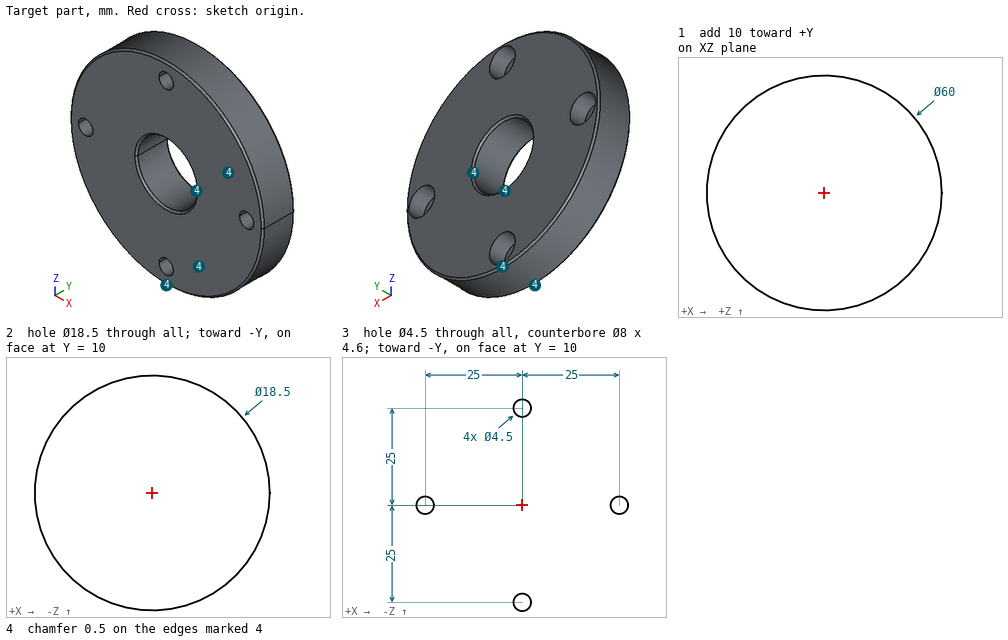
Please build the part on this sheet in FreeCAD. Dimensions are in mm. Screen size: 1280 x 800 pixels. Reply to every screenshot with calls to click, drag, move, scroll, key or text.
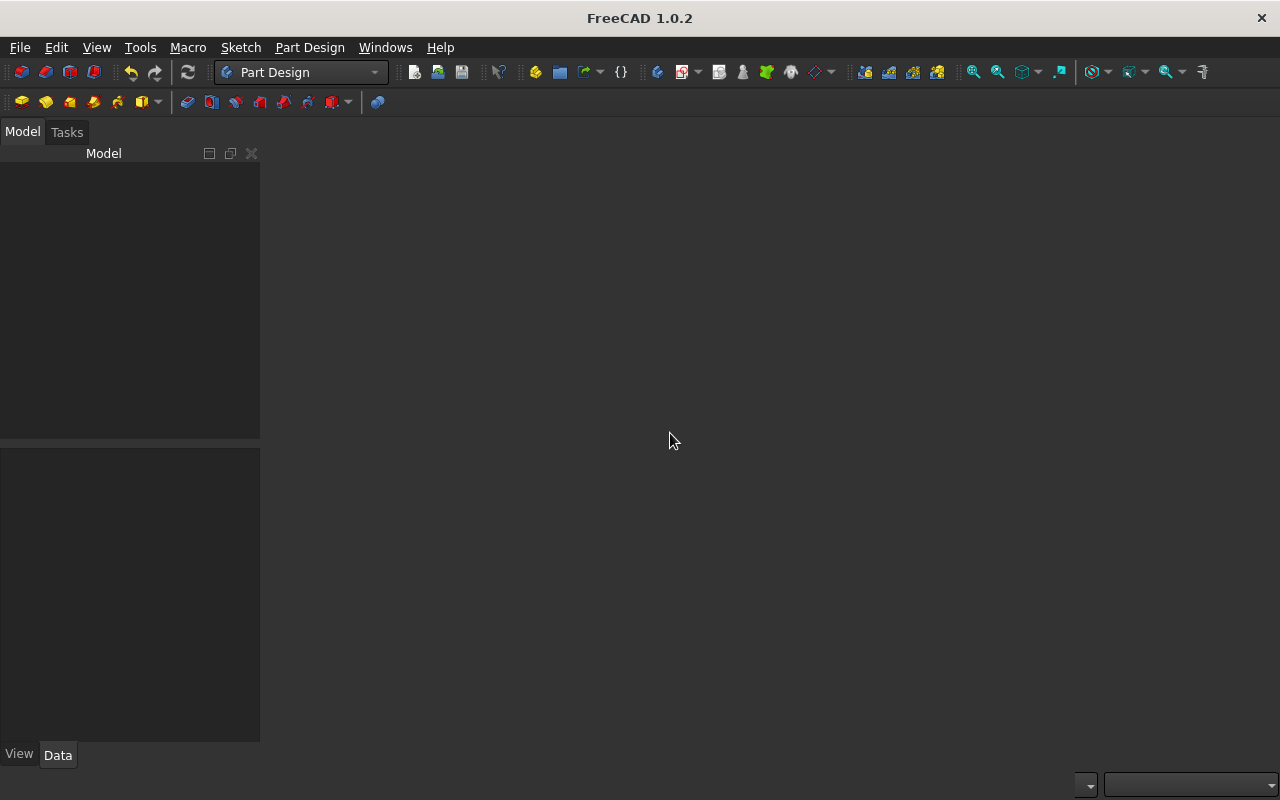
key(ctrl+n)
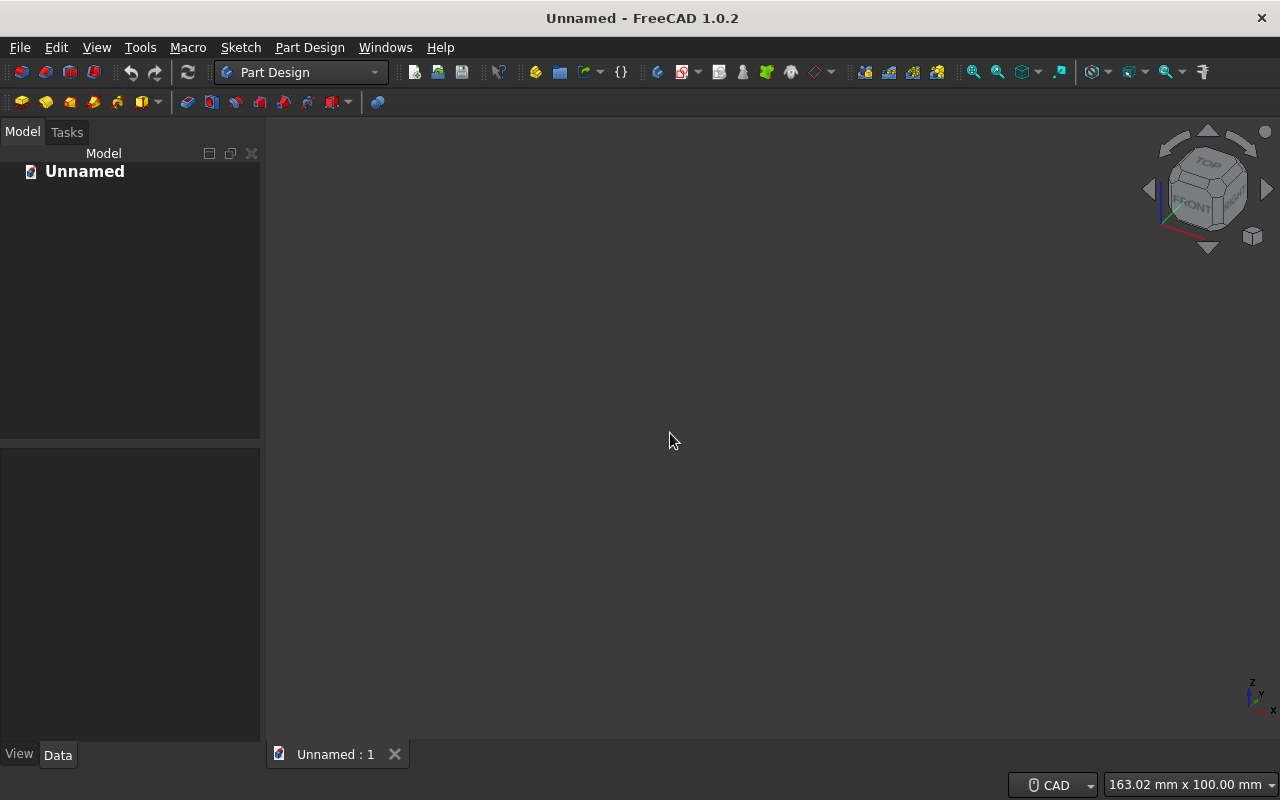
click(682, 72)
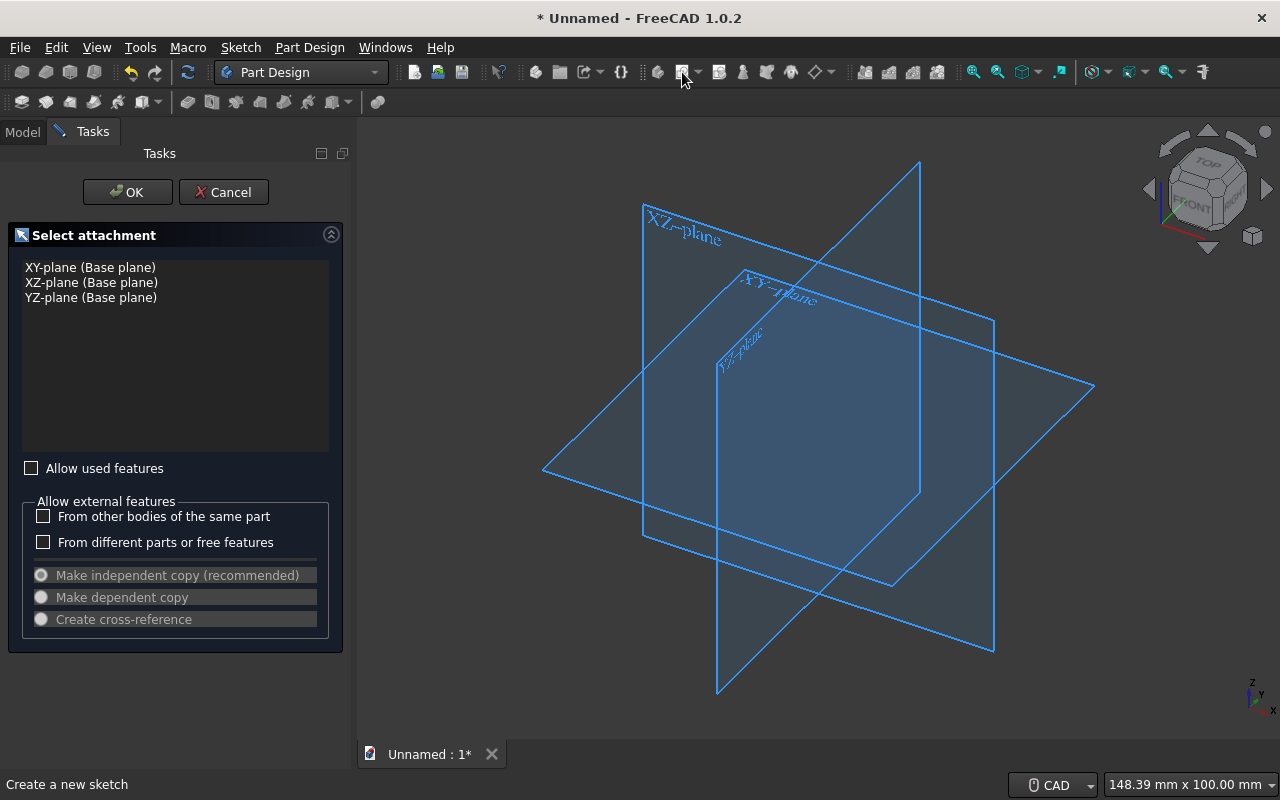
click(82, 282)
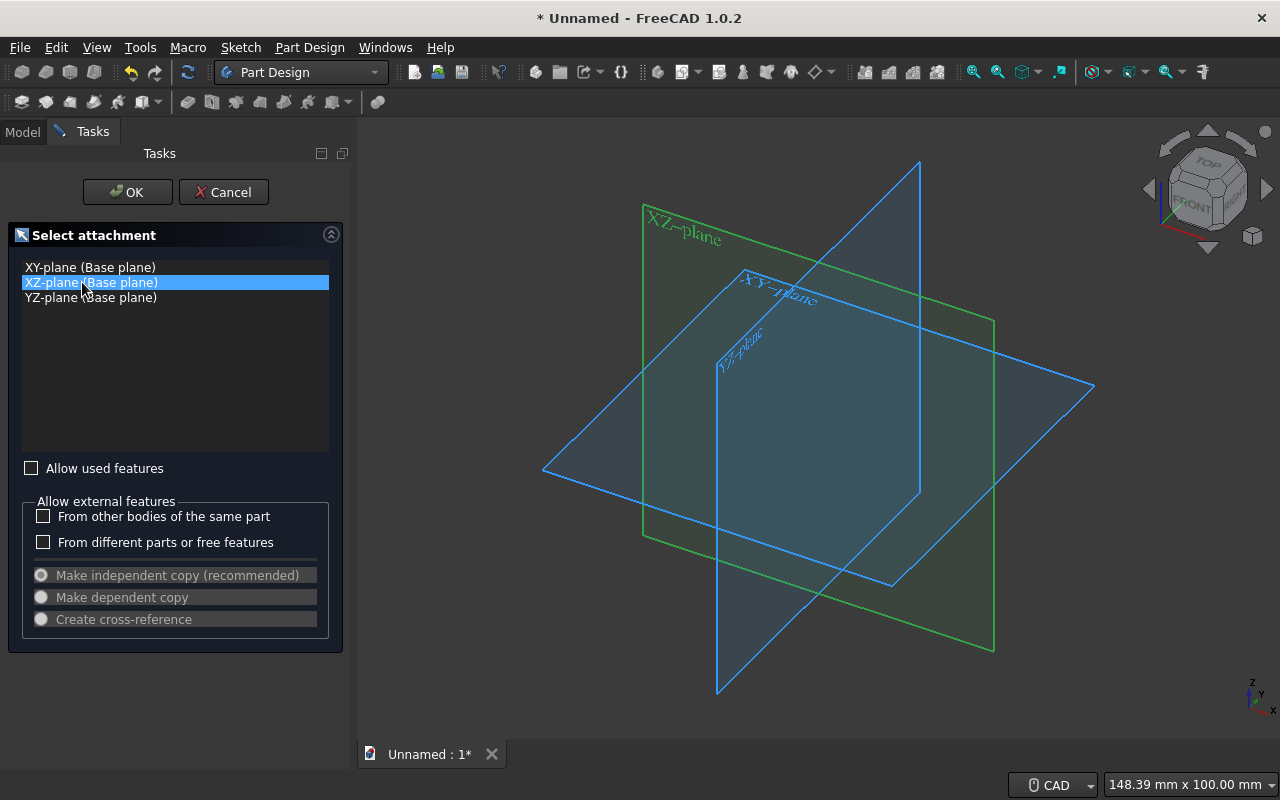
click(128, 192)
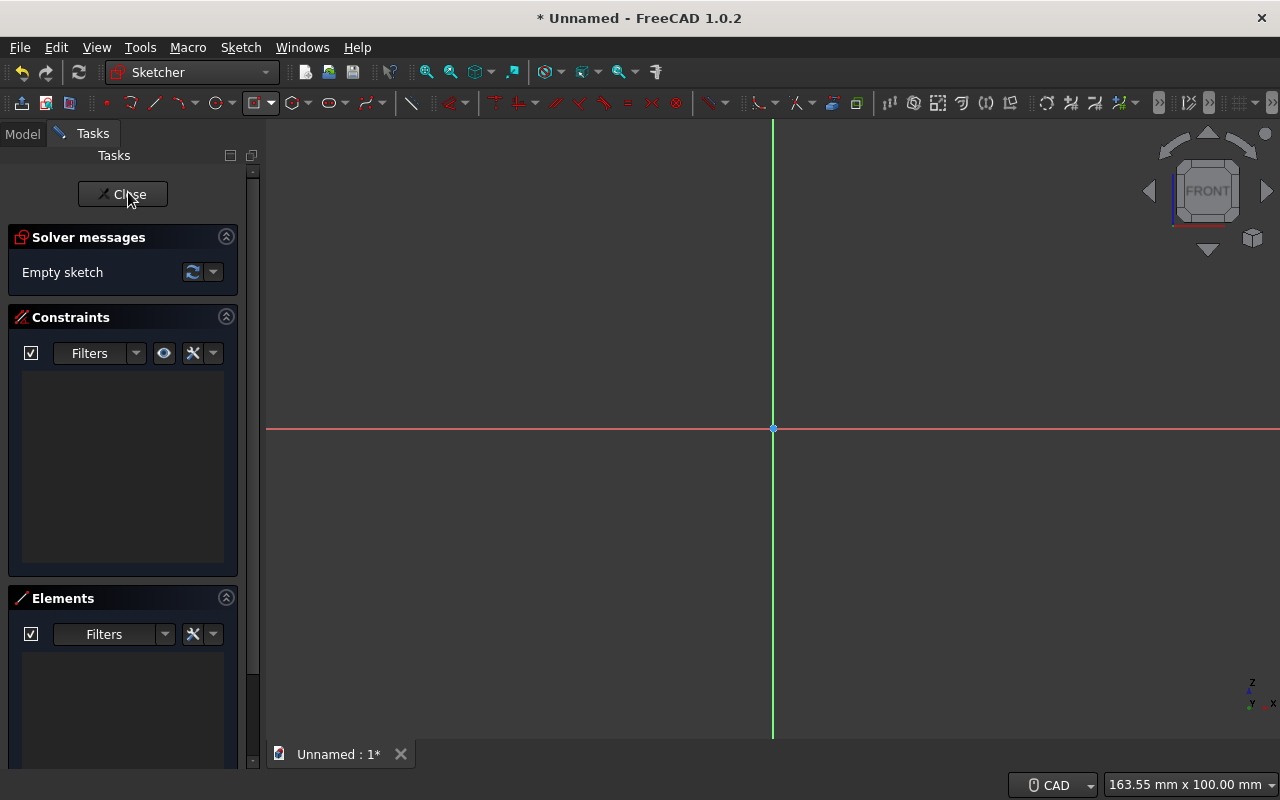
key(g)
key(c)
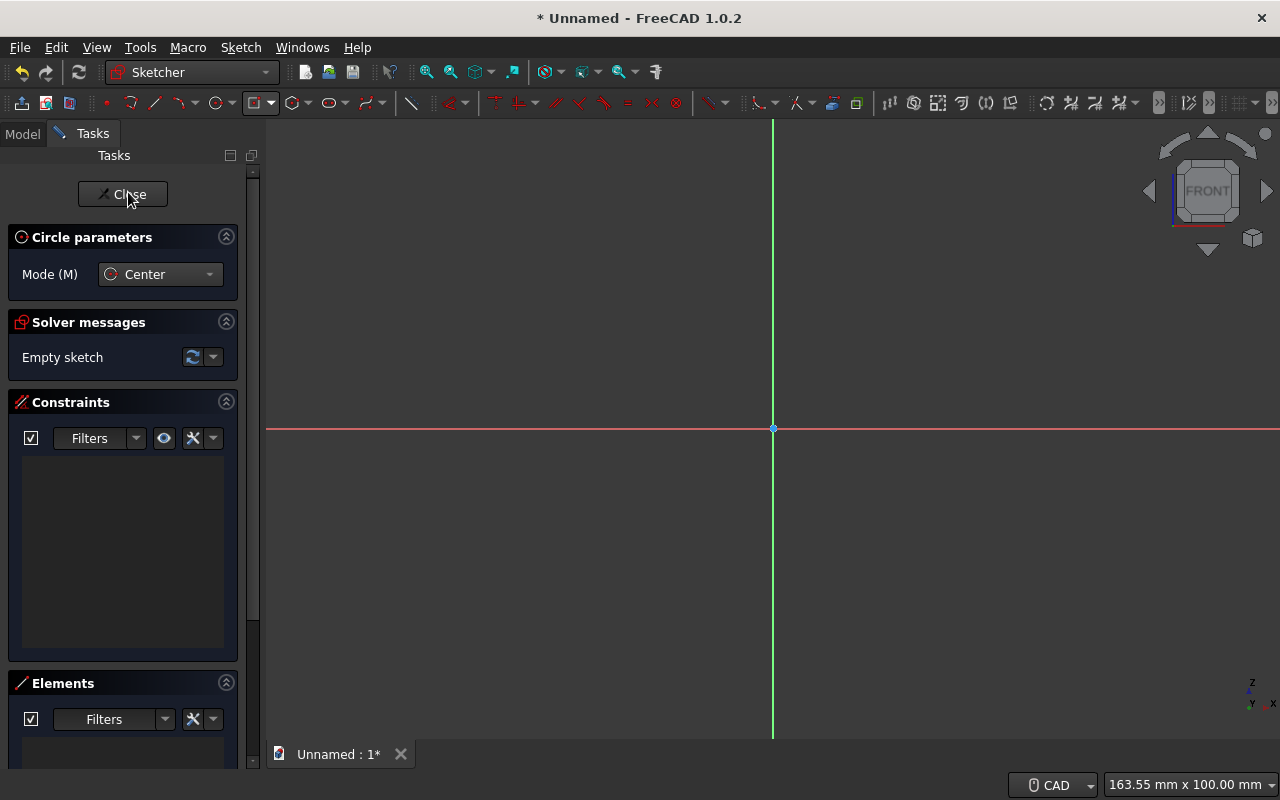
click(773, 429)
click(905, 297)
key(Escape)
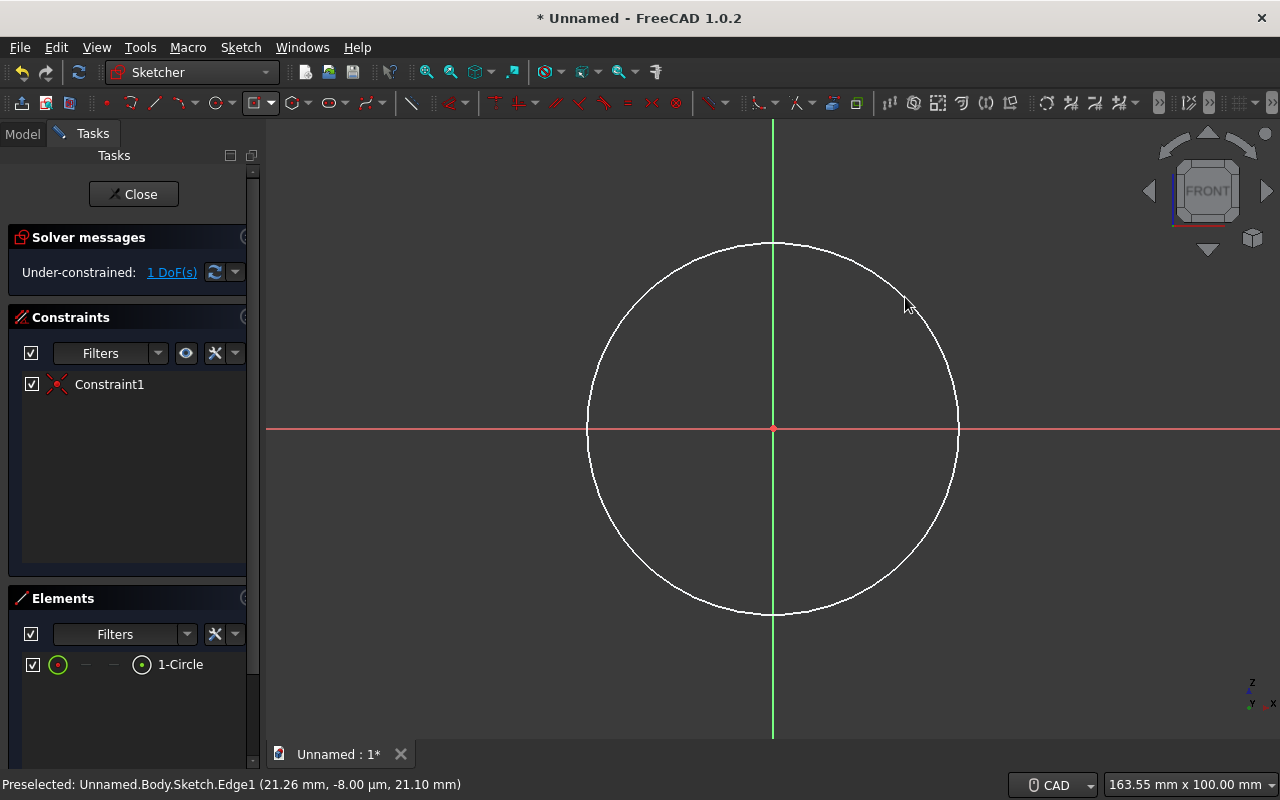
key(d)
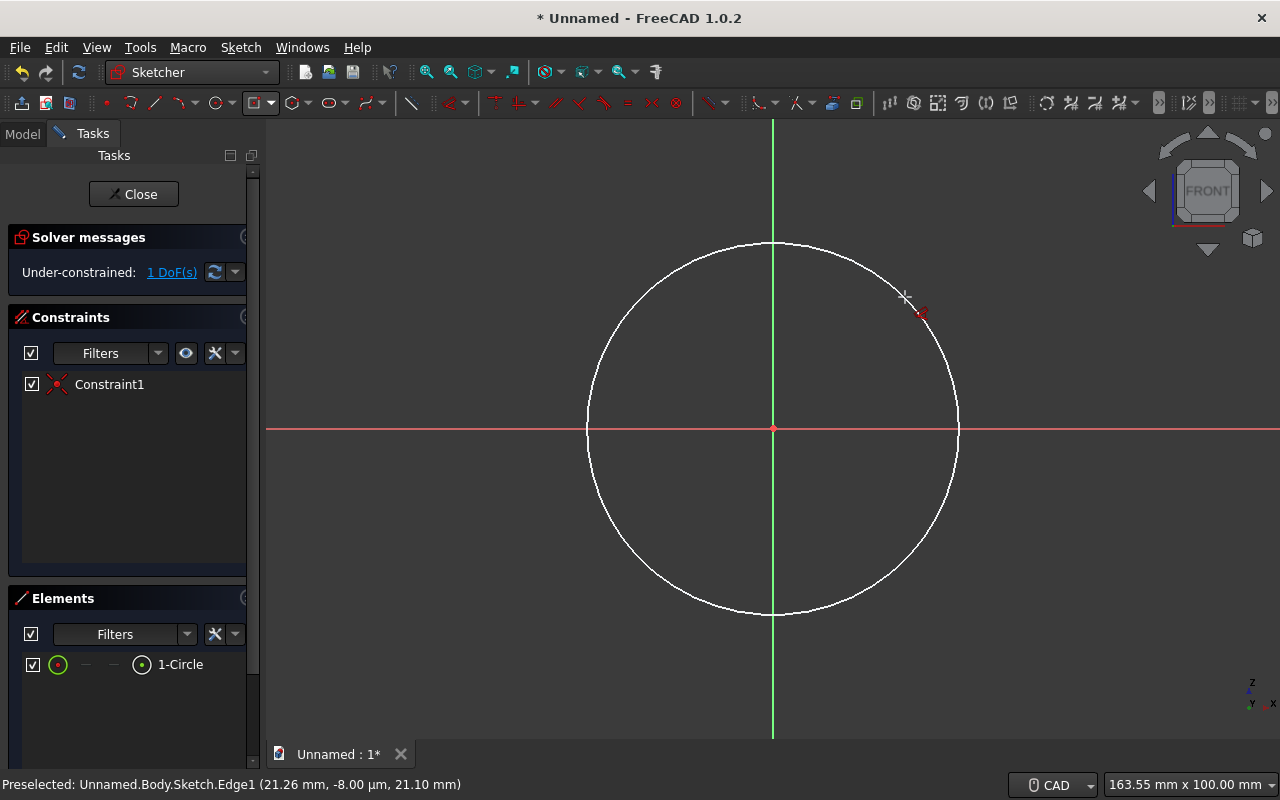
click(904, 297)
click(927, 274)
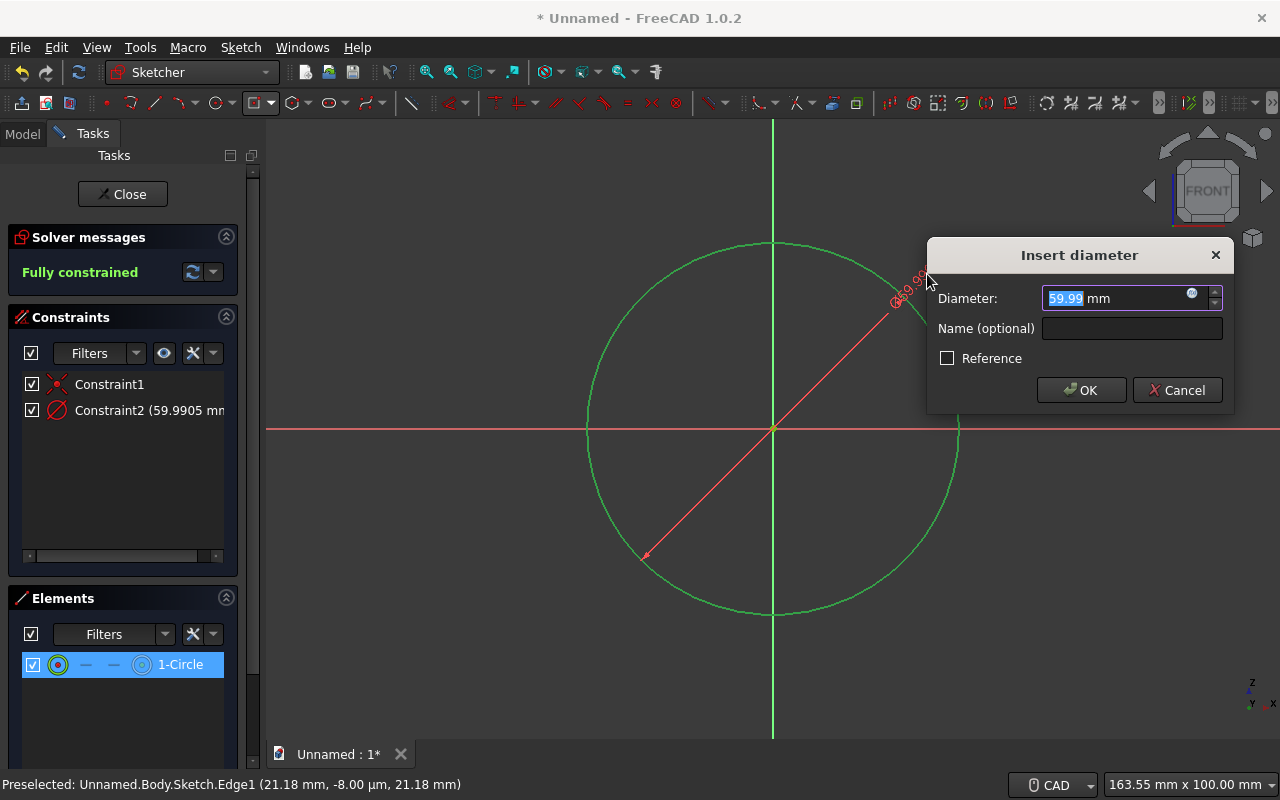
text(60)
key(Return)
key(Escape)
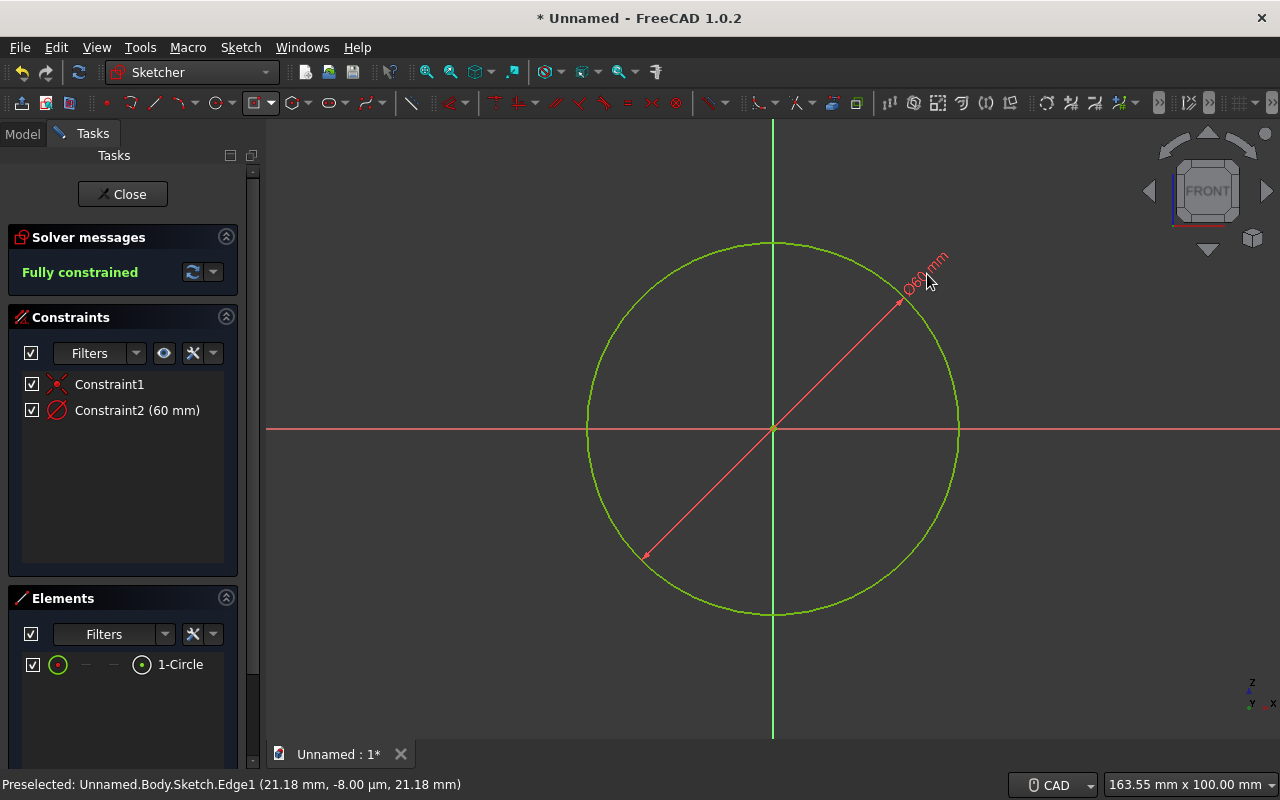
click(123, 194)